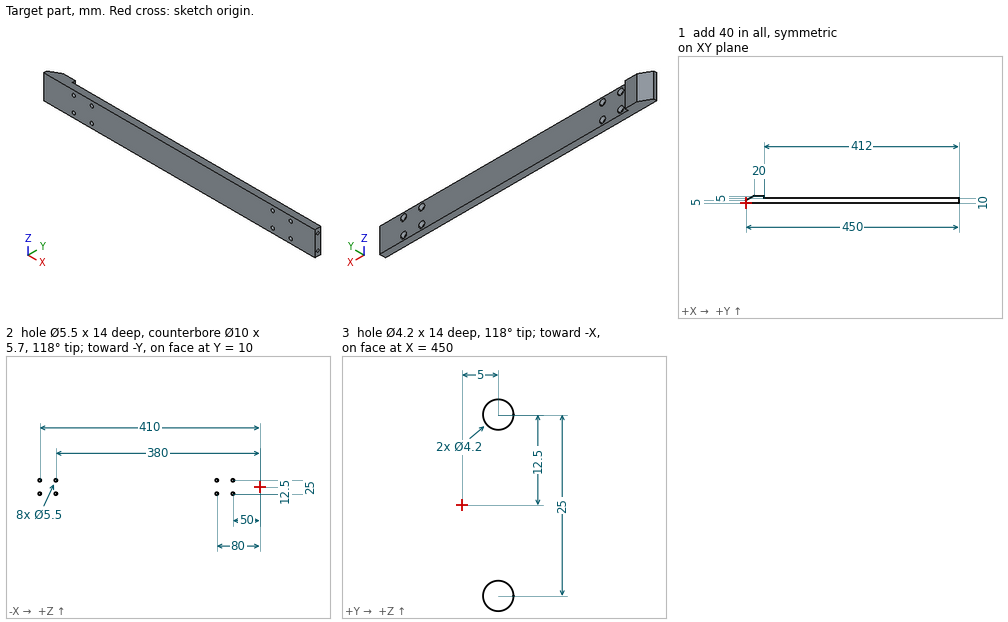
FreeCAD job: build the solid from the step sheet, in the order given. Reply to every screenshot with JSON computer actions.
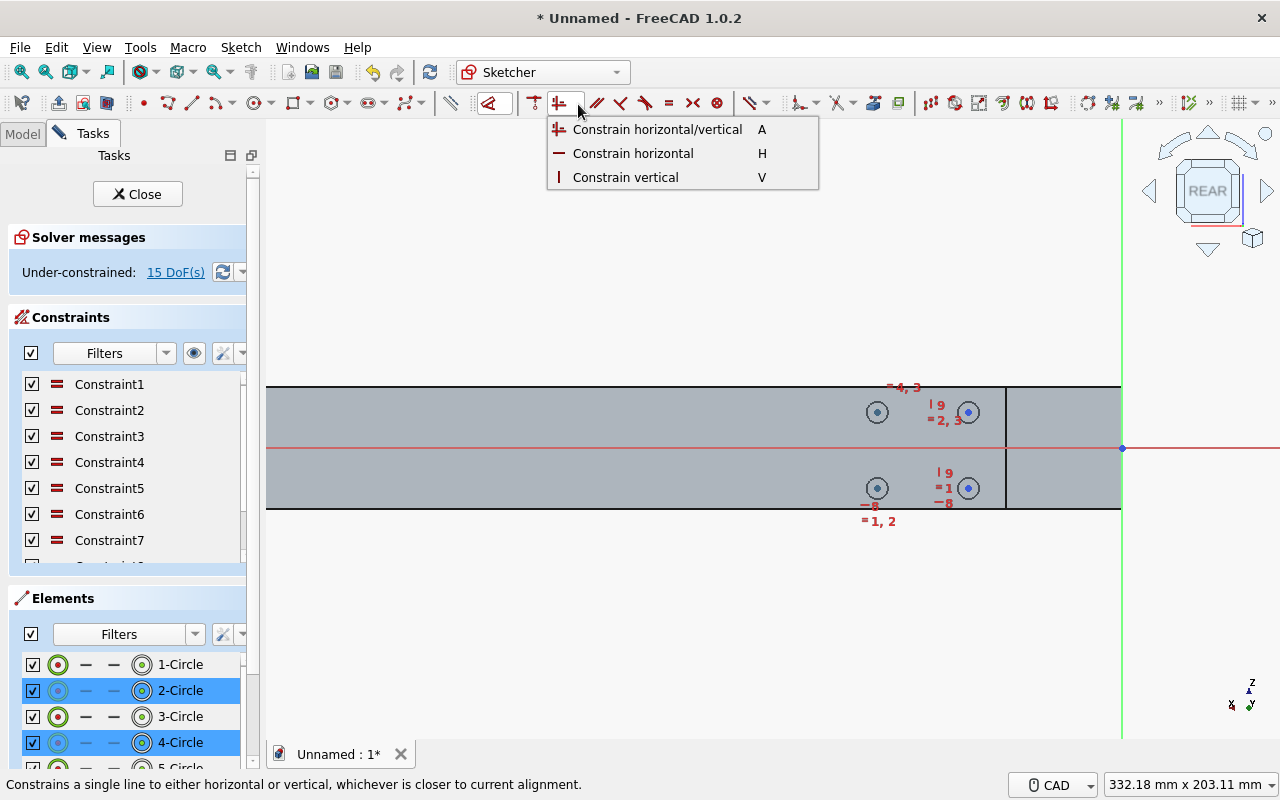
{"action": "left_click", "coordinate": [683, 177]}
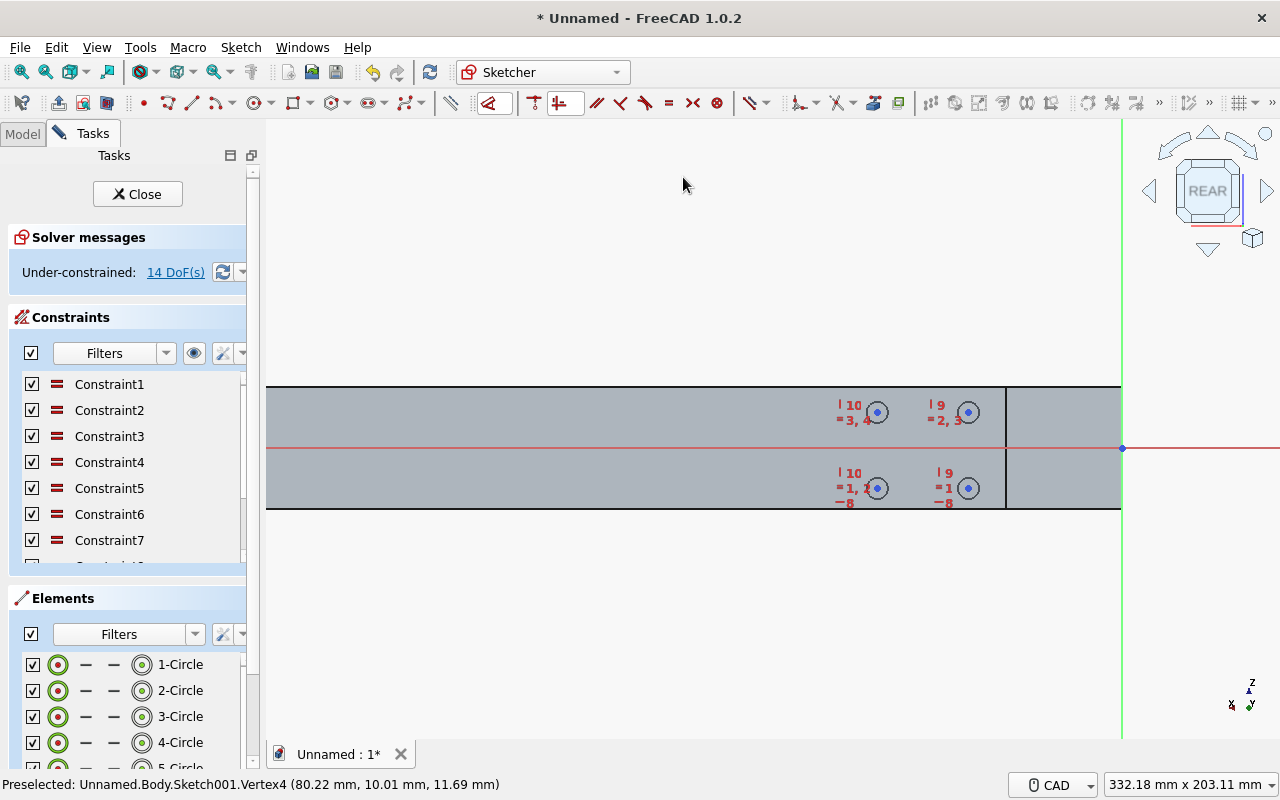
{"action": "left_click", "coordinate": [969, 412]}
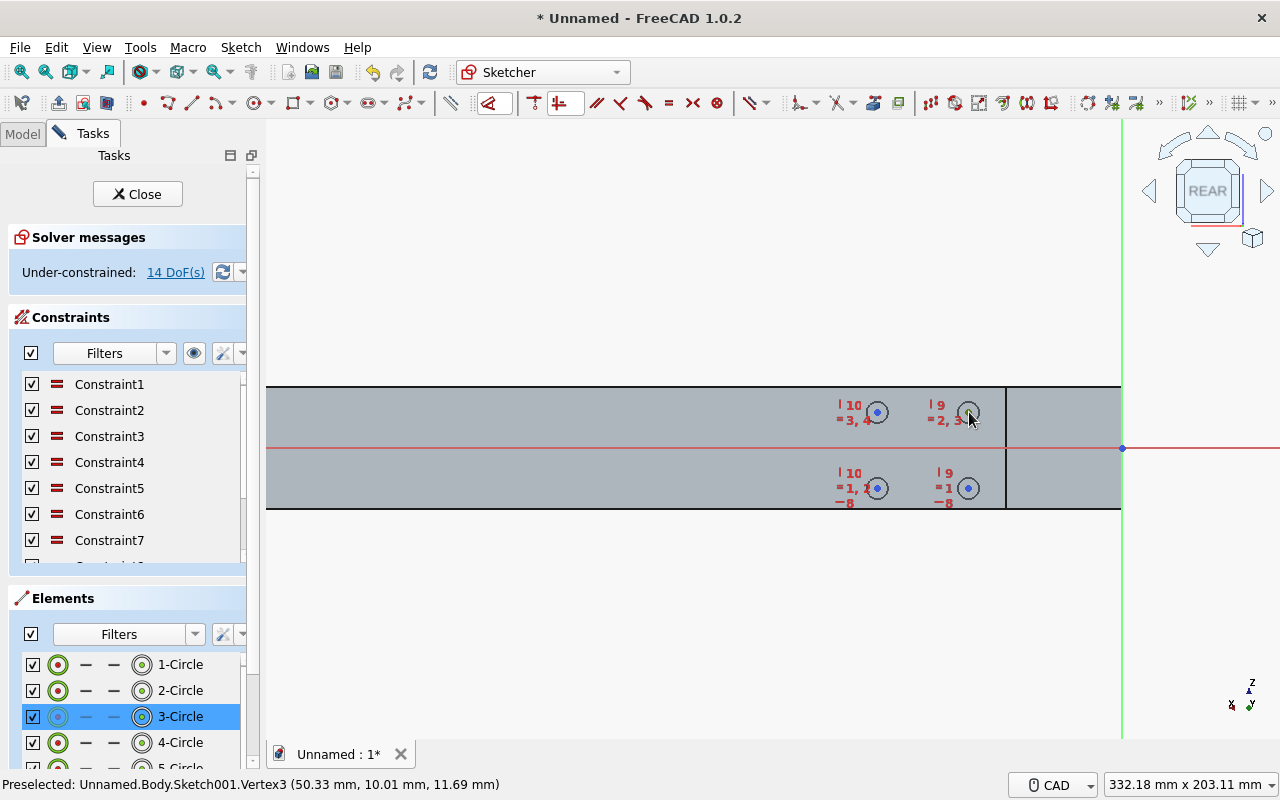
{"action": "left_click", "coordinate": [877, 412]}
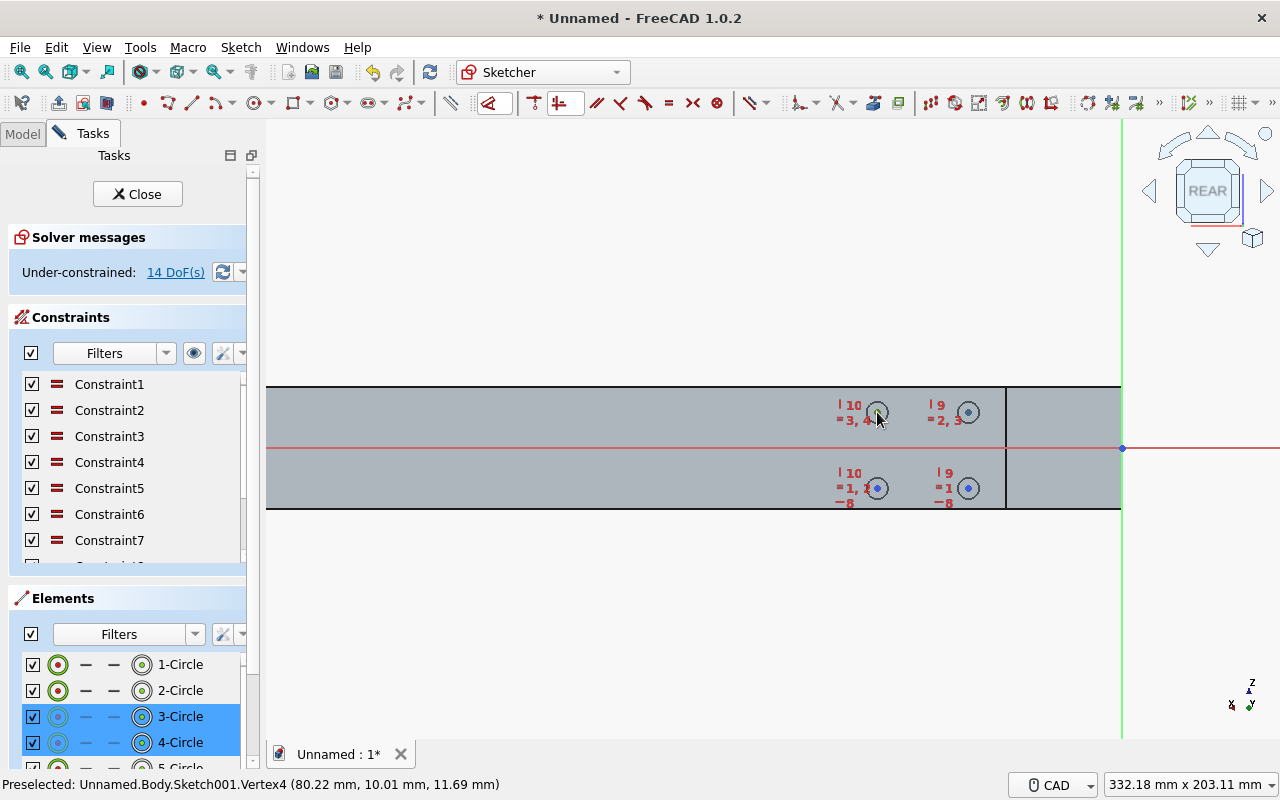
{"action": "left_click", "coordinate": [578, 104]}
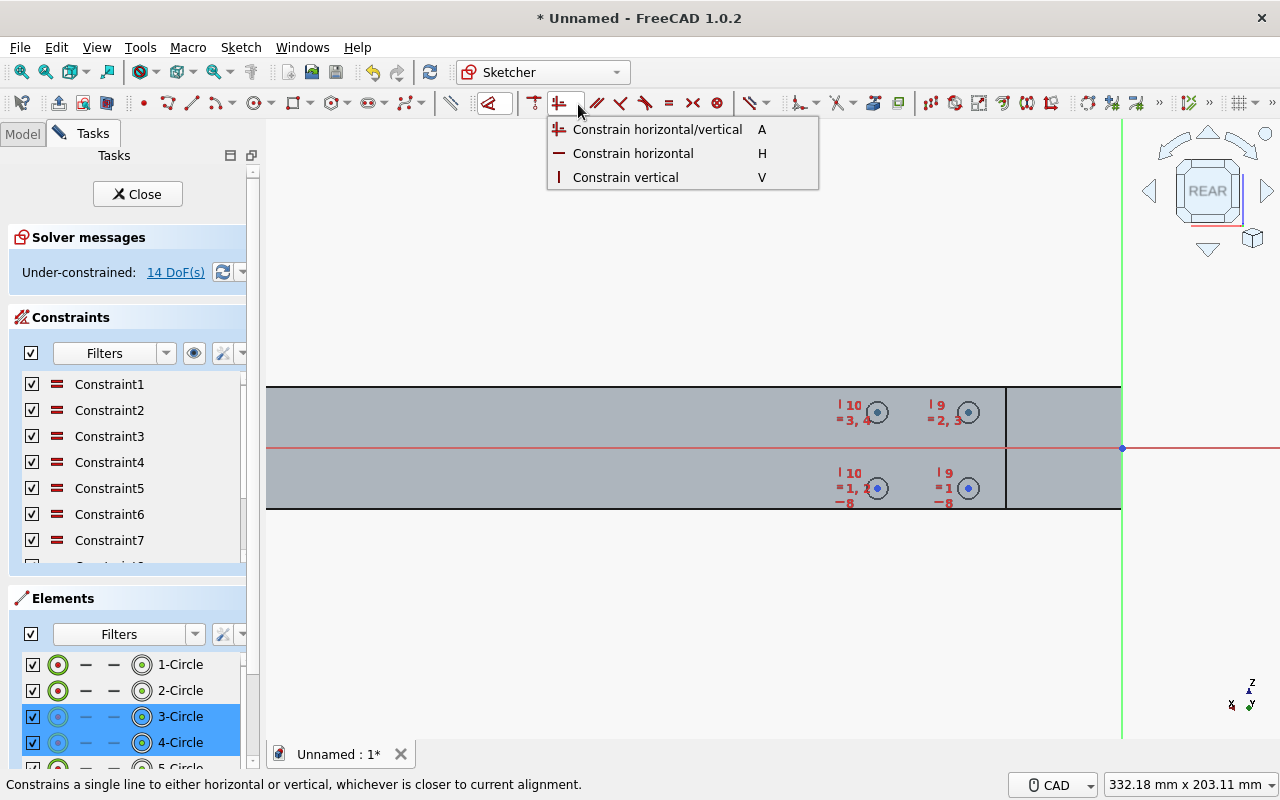
{"action": "left_click", "coordinate": [683, 153]}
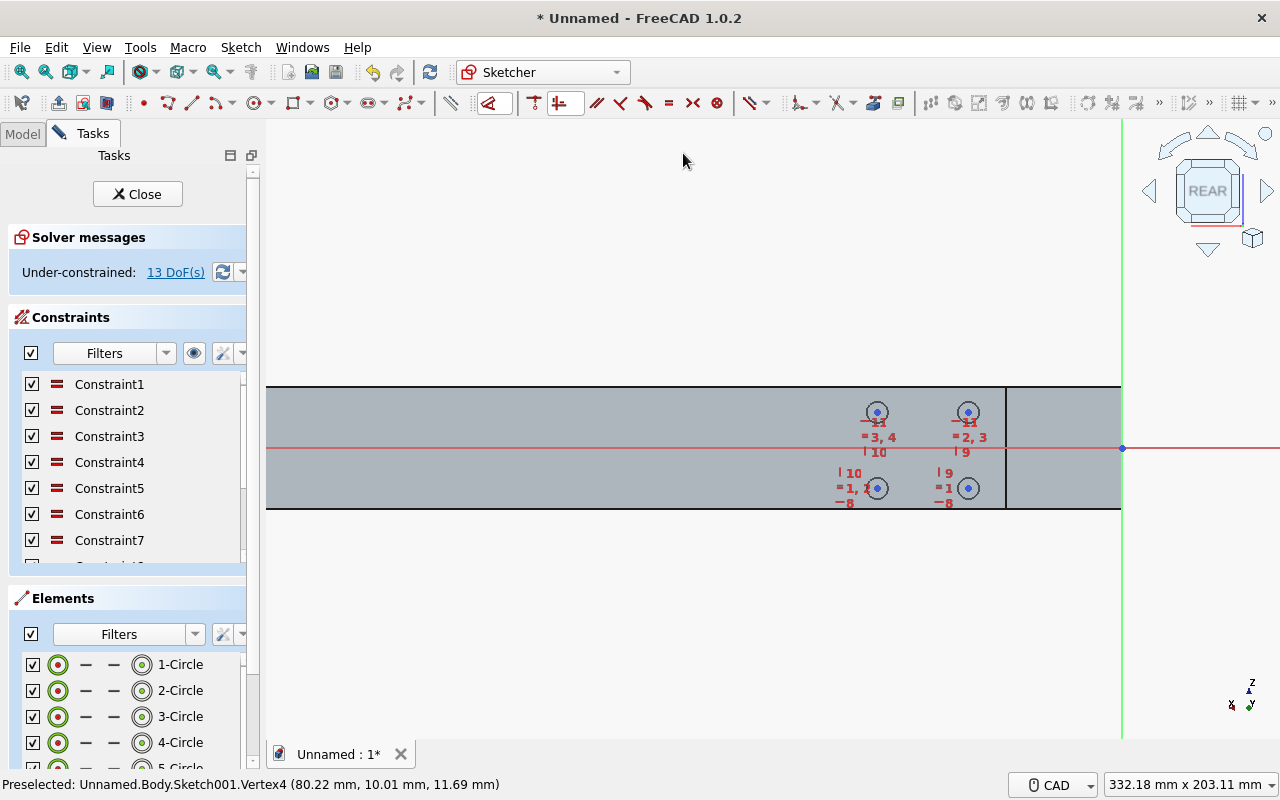
{"action": "left_click", "coordinate": [877, 412]}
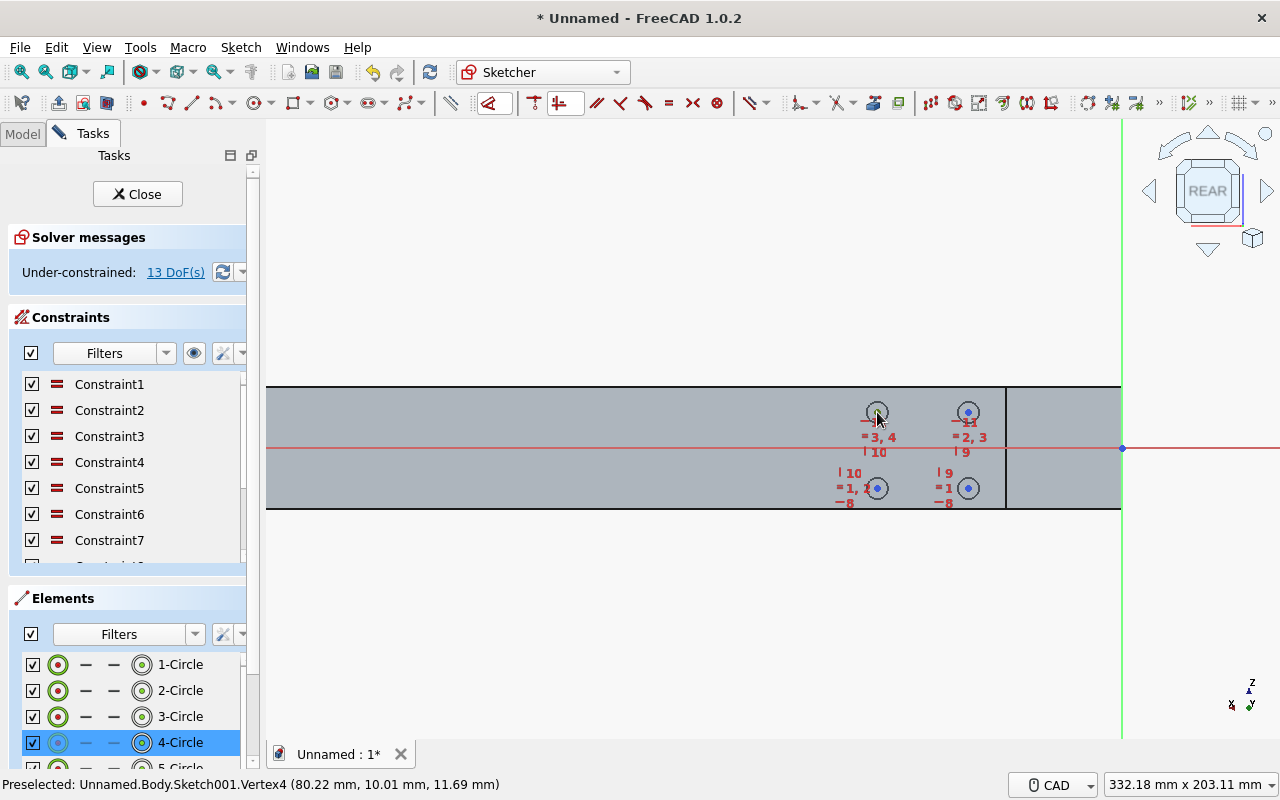
{"action": "scroll", "coordinate": [878, 413], "scroll_direction": "down", "scroll_amount": 4}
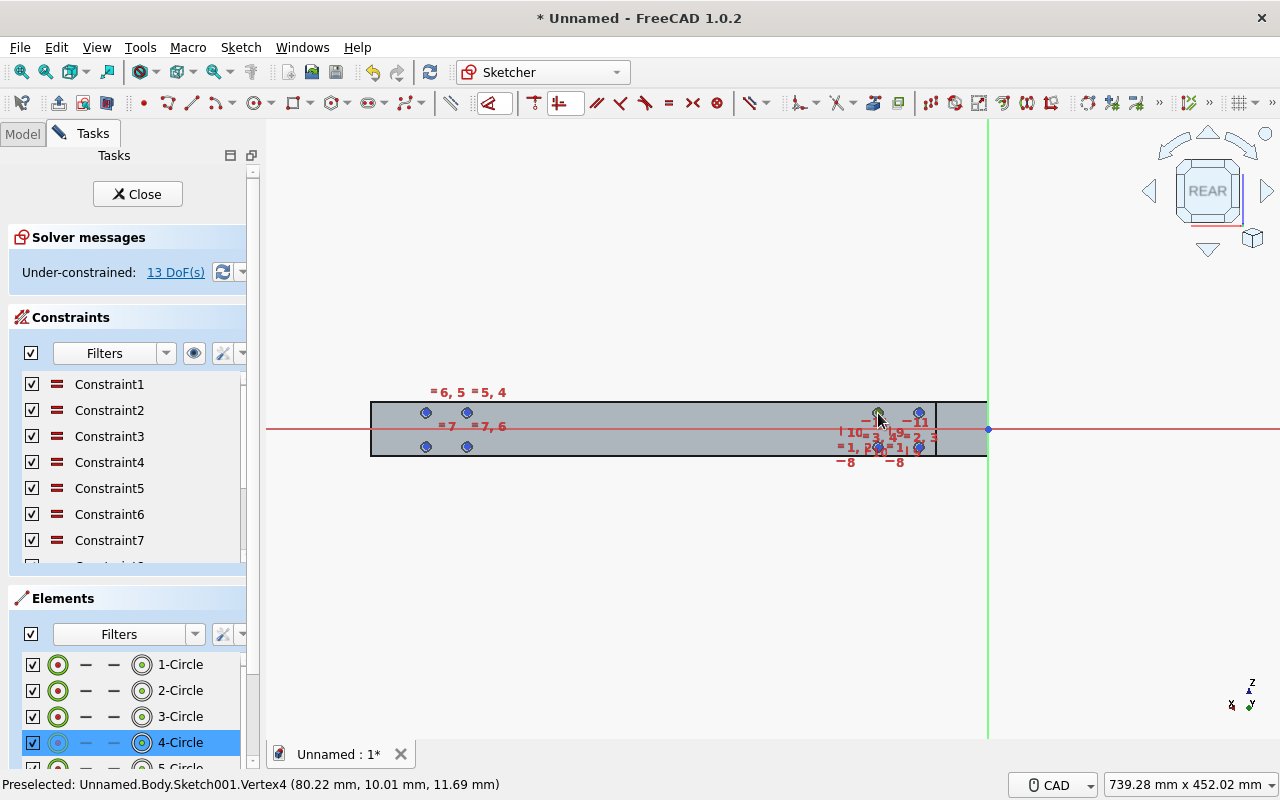
{"action": "left_click", "coordinate": [467, 413]}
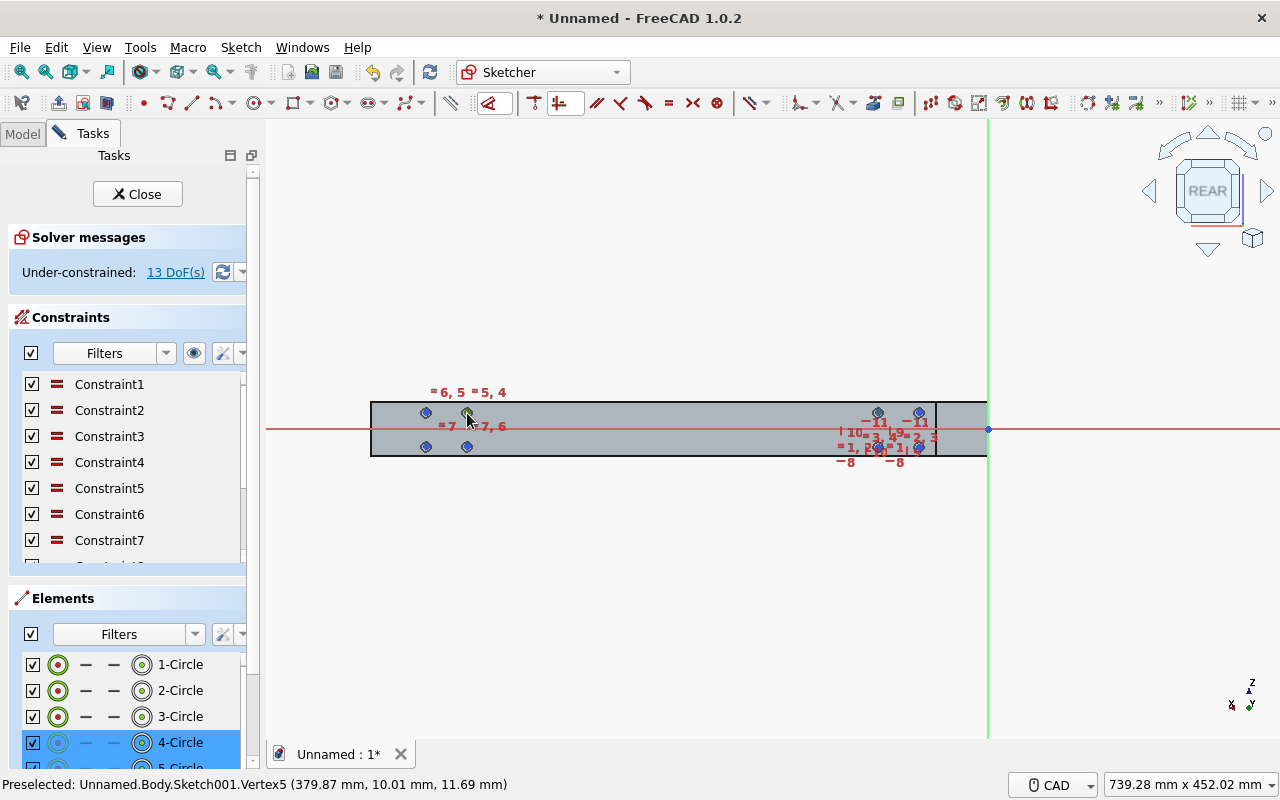
{"action": "left_click", "coordinate": [578, 104]}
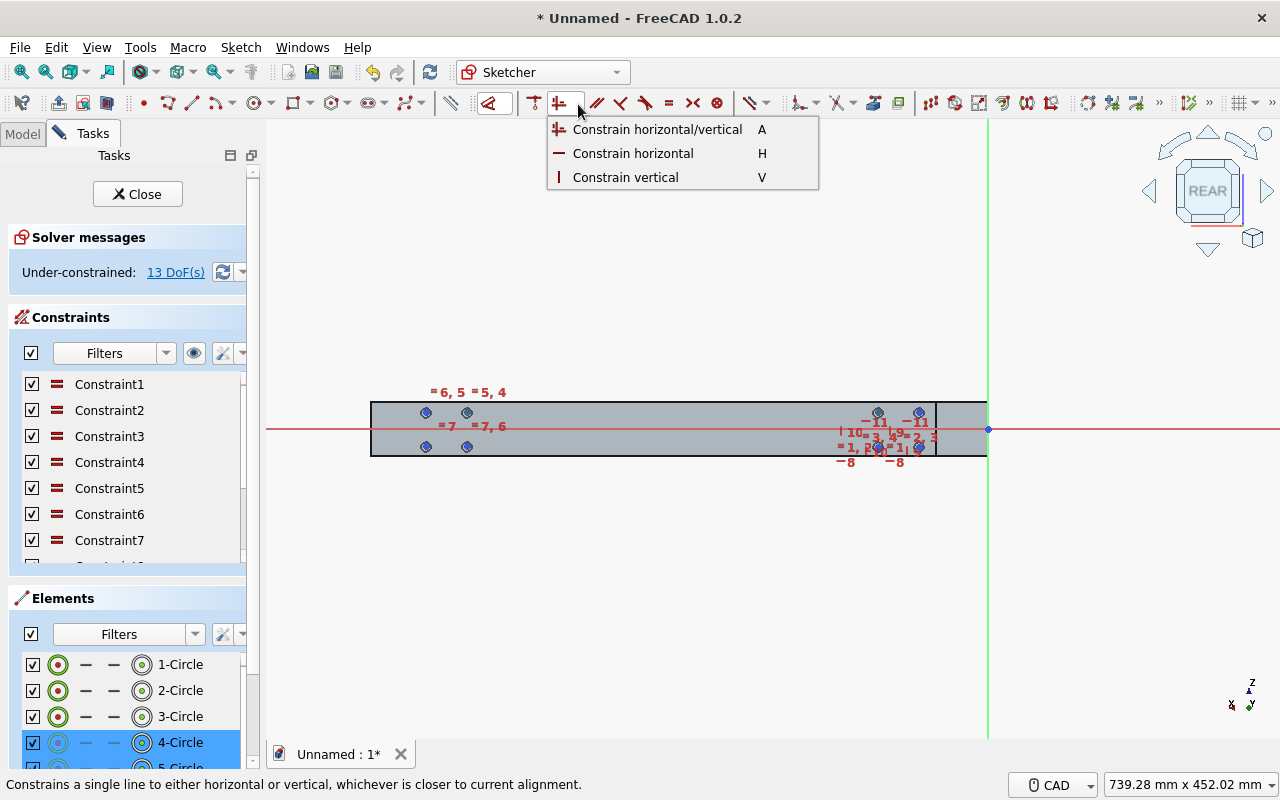
{"action": "left_click", "coordinate": [683, 153]}